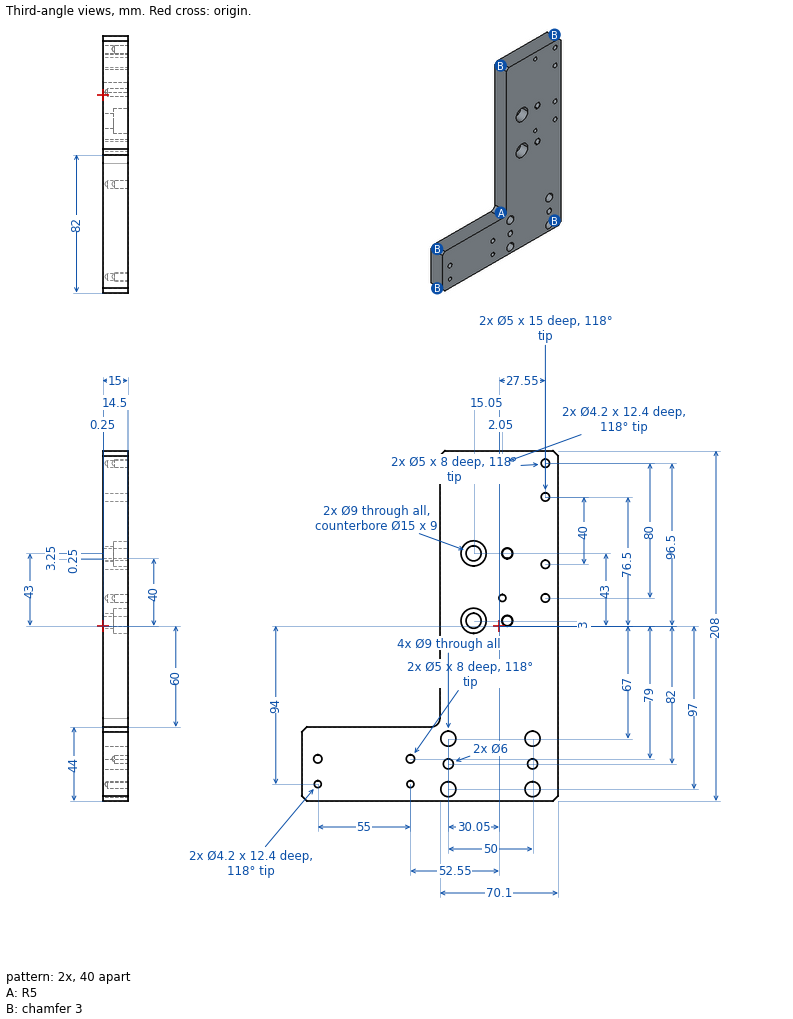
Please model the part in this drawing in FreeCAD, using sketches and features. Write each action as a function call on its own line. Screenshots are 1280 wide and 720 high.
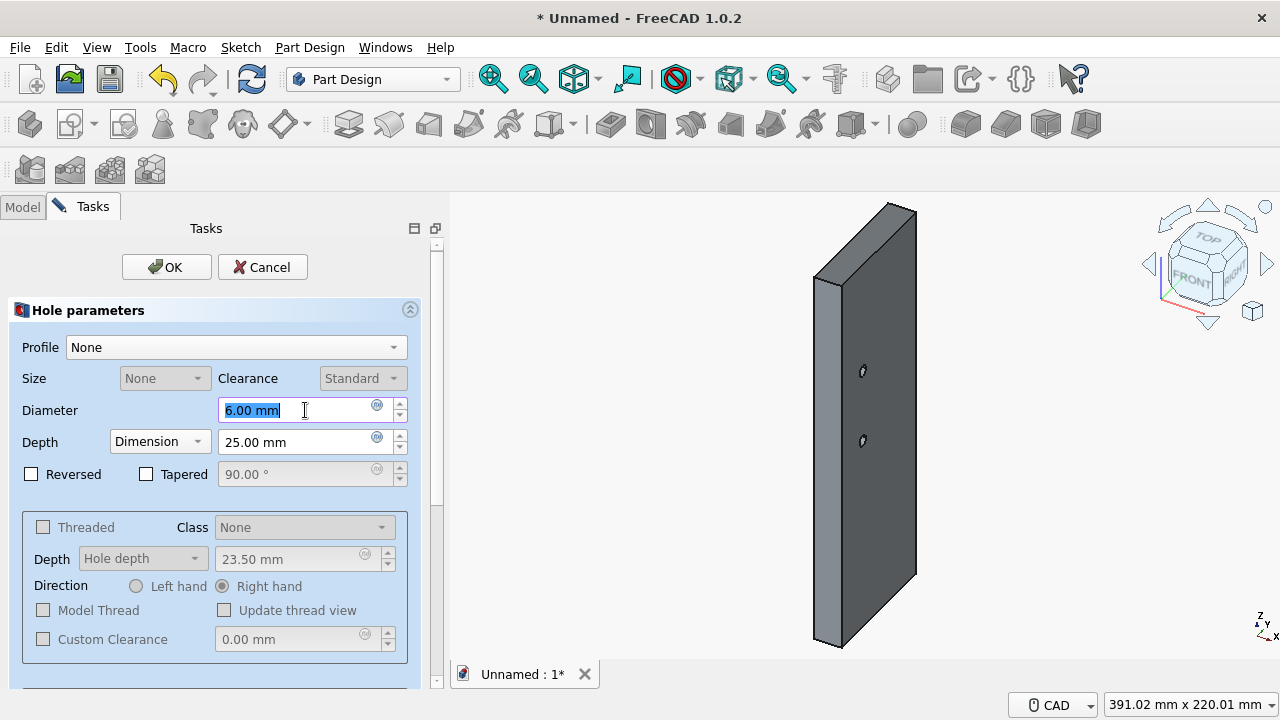
text(9)
key(Tab)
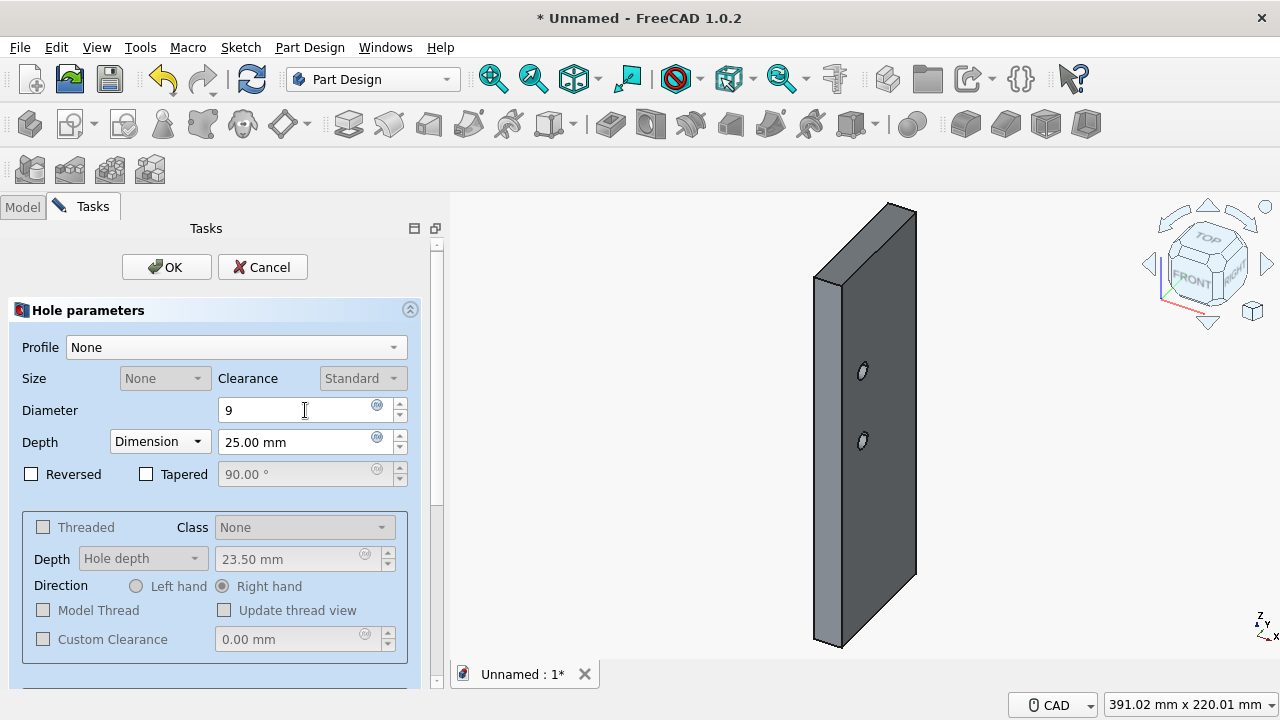
click(161, 442)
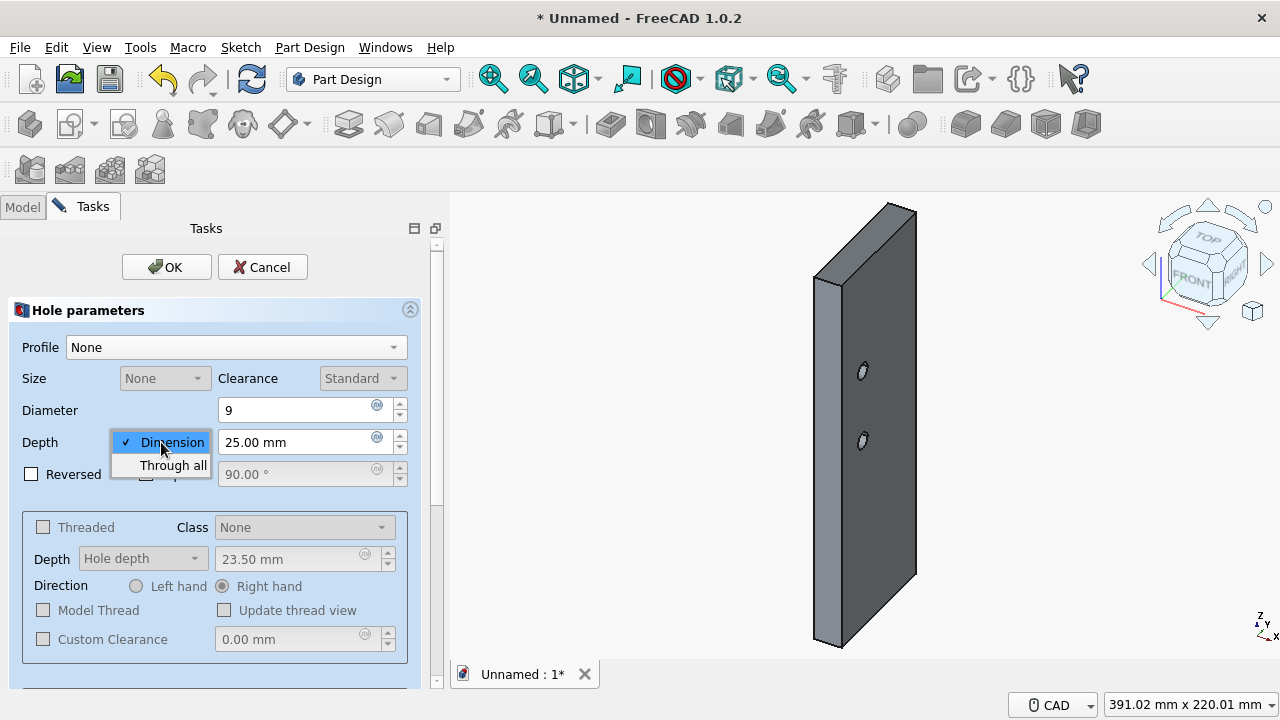
click(160, 466)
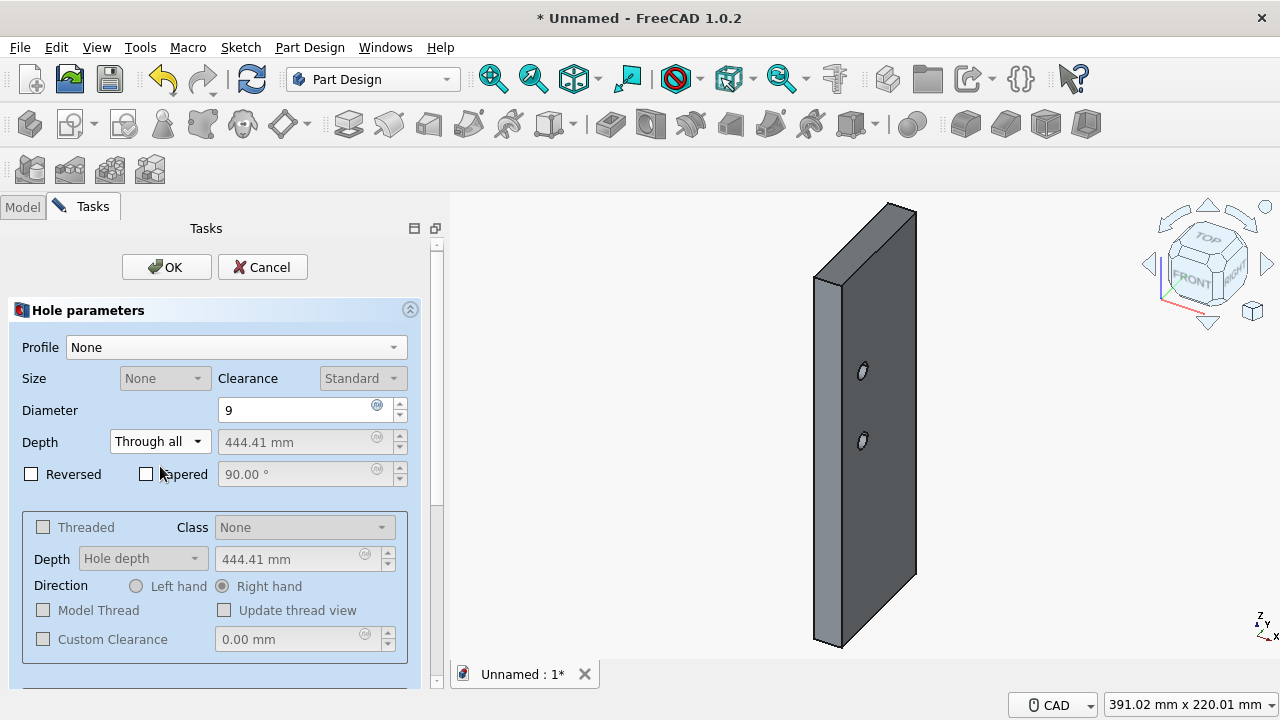
scroll(437, 463, down, 2)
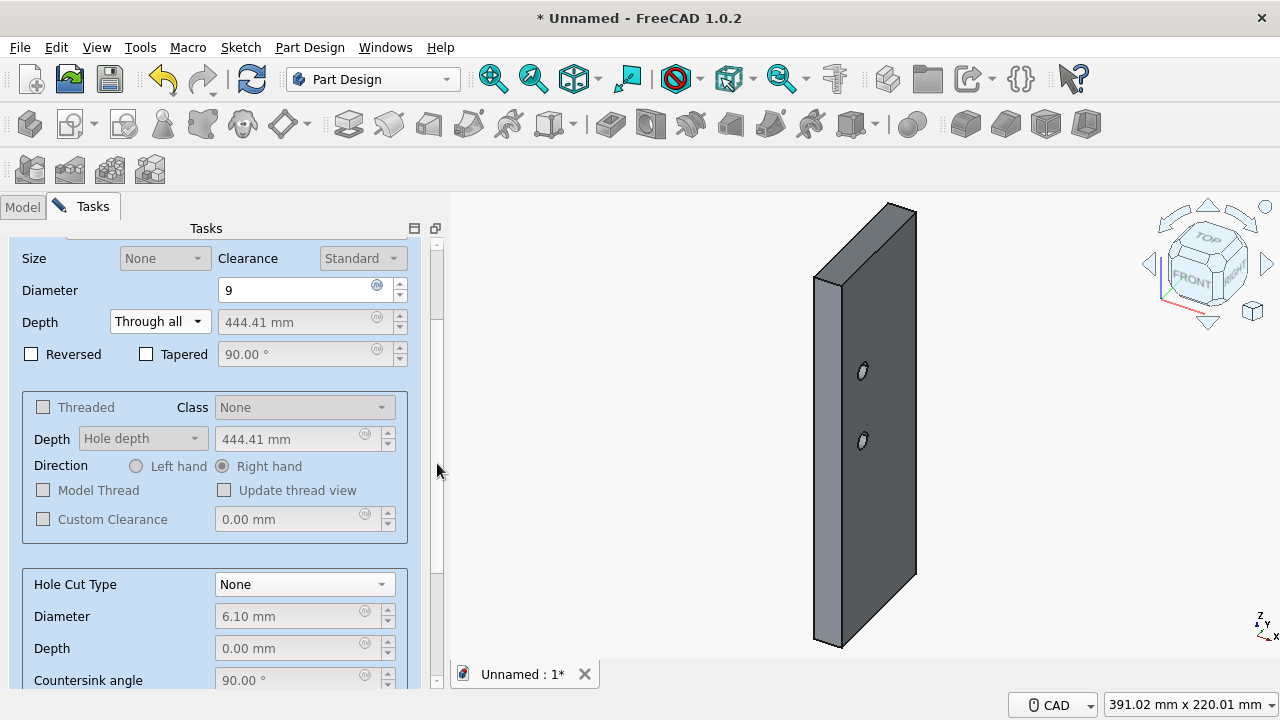
click(306, 584)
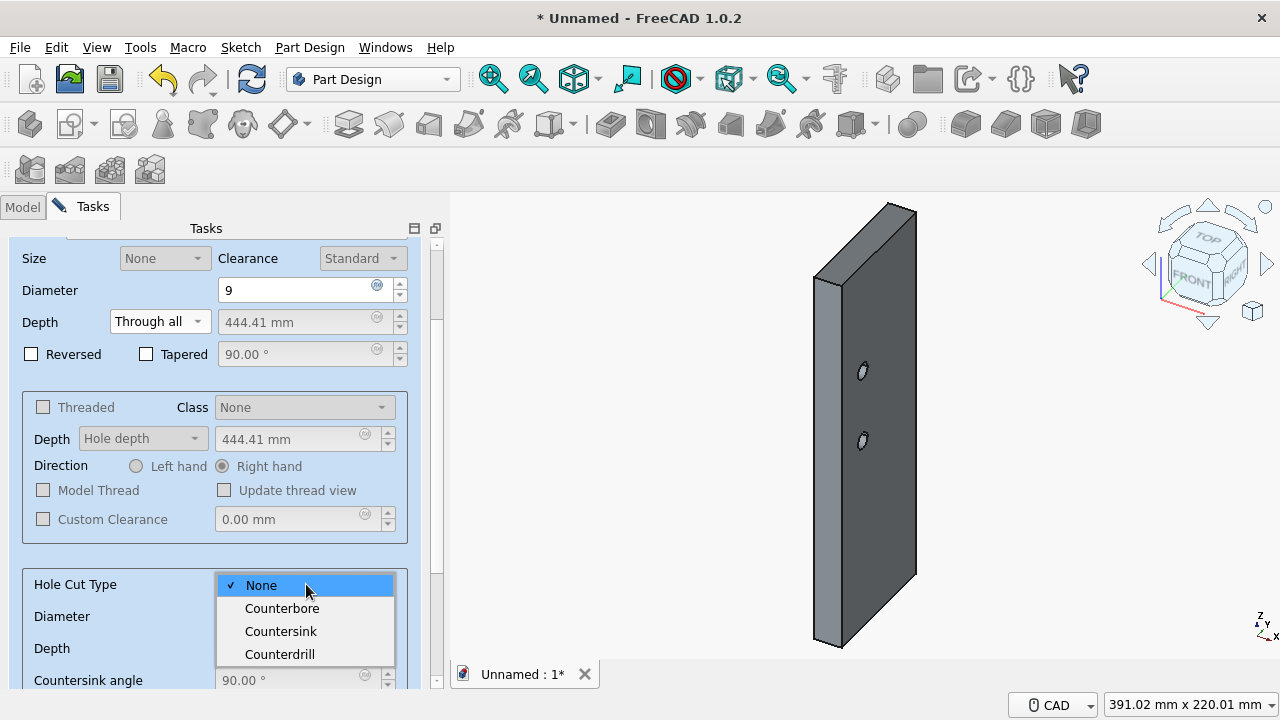
click(304, 608)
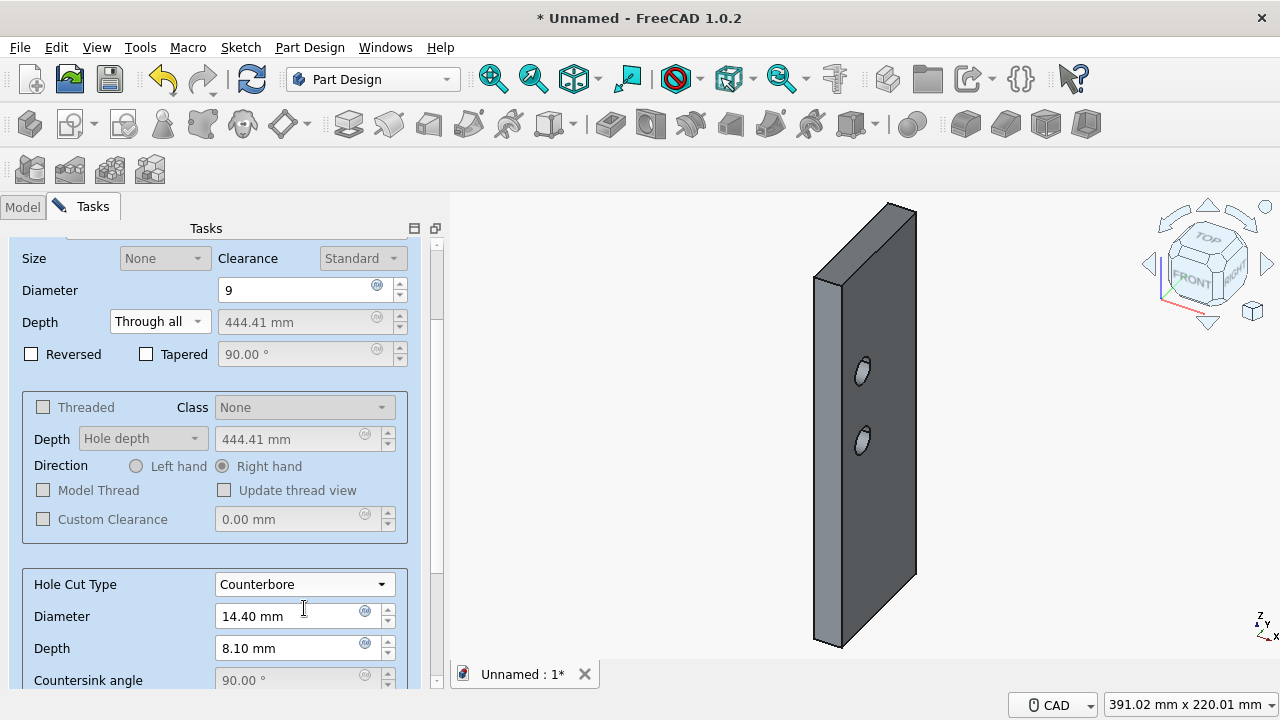
triple_click(298, 616)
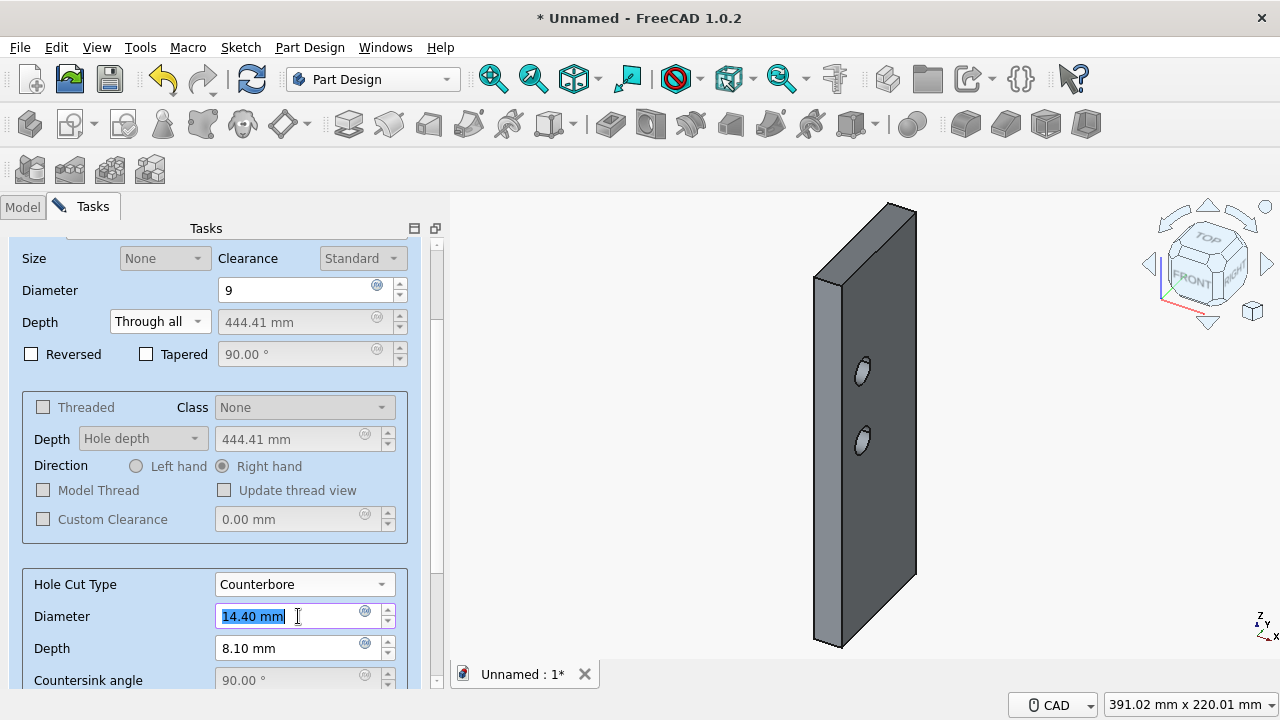
text(15)
key(Tab)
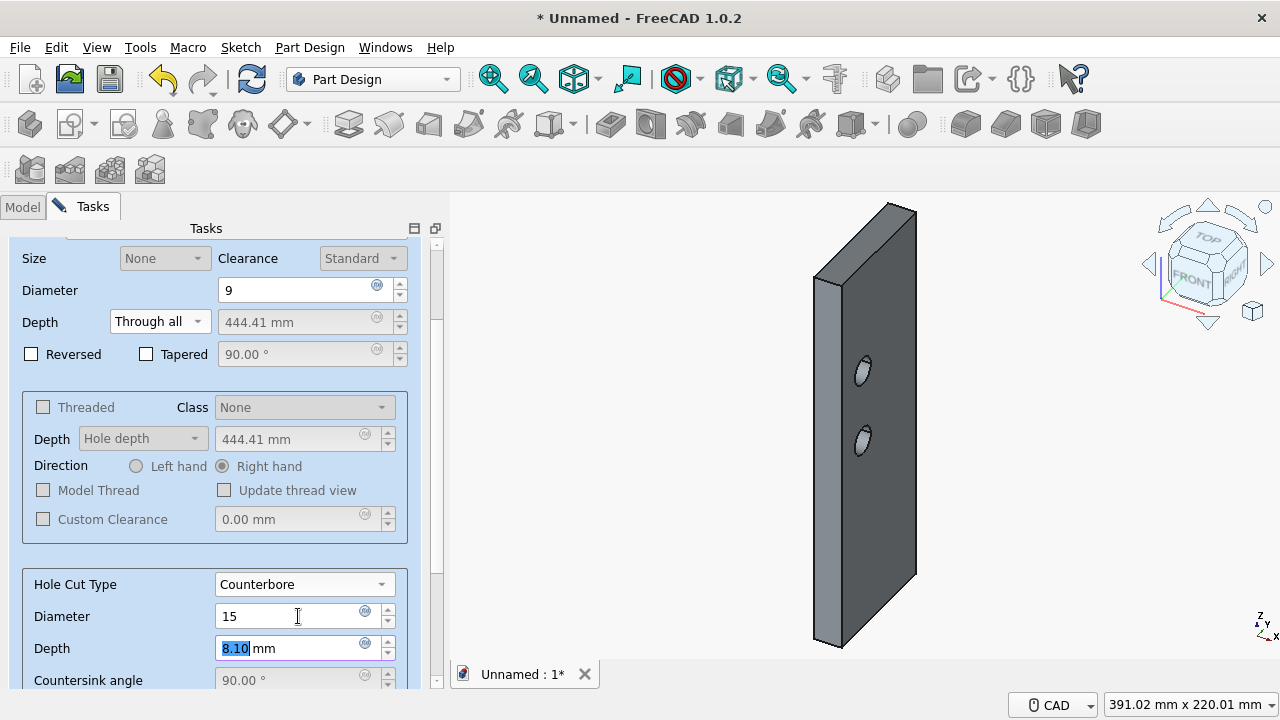
text(9)
key(Tab)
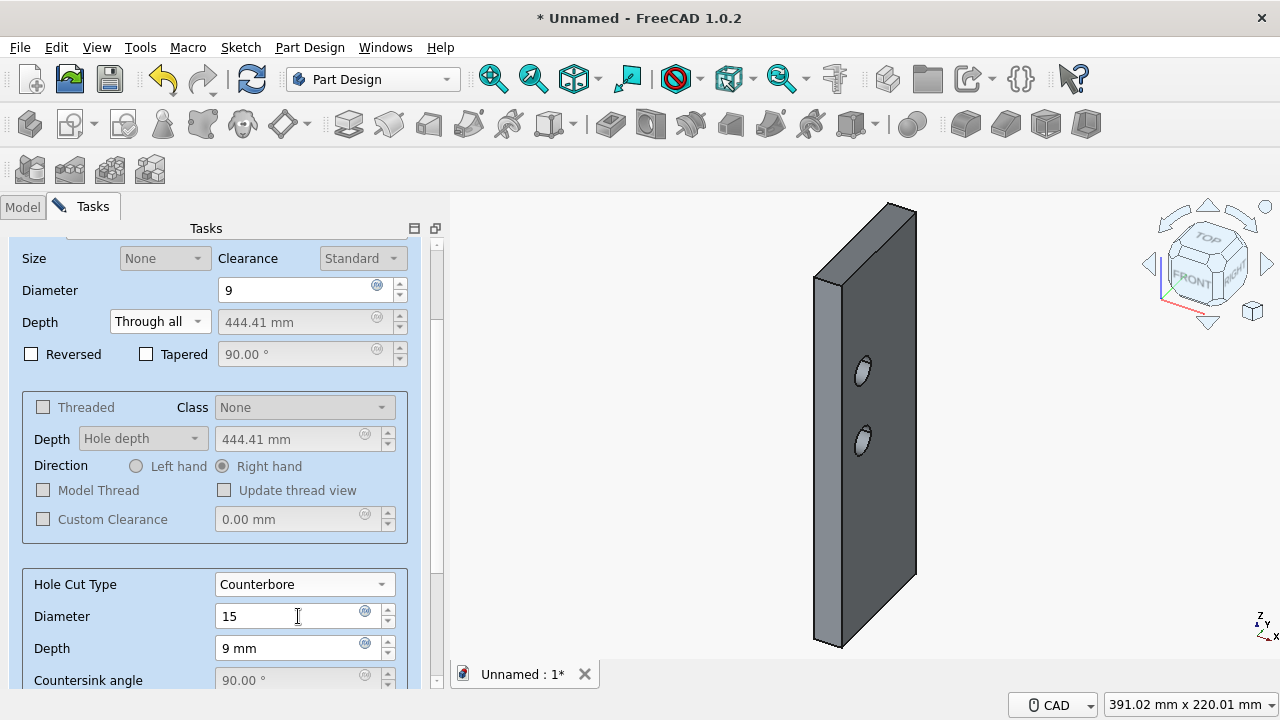
scroll(437, 463, up, 3)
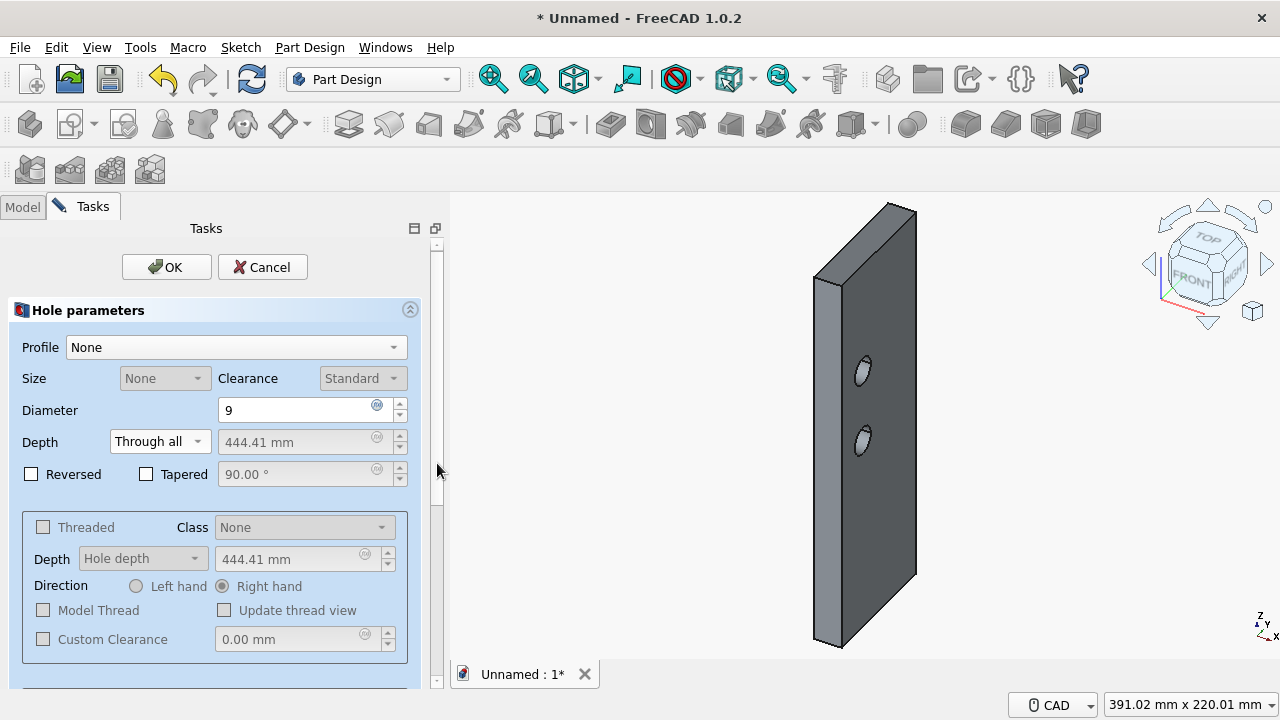
click(167, 267)